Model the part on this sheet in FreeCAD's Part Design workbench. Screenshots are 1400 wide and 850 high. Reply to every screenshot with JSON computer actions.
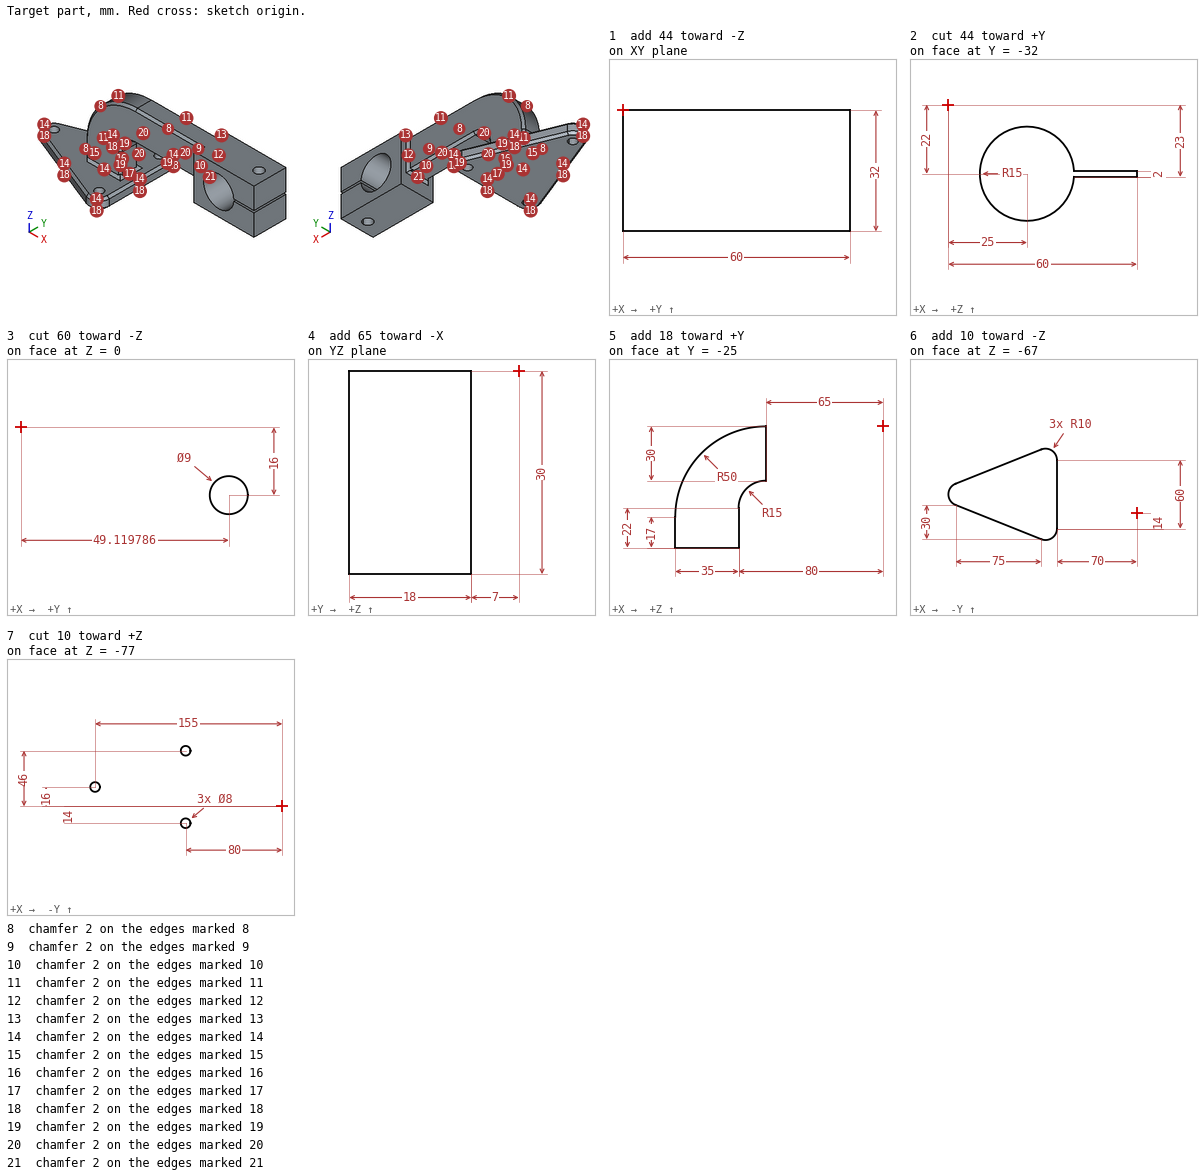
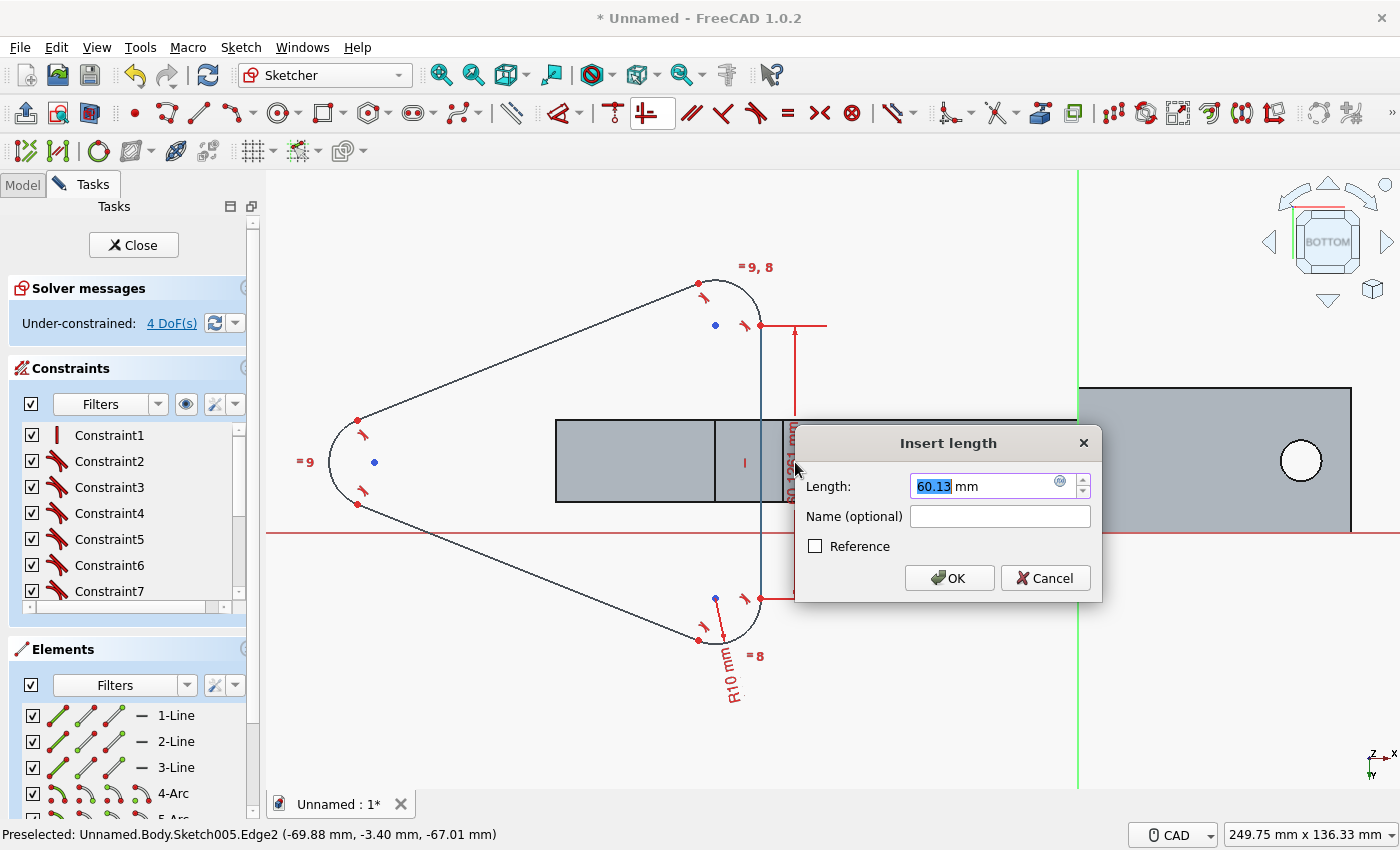
{"action": "type", "text": "60"}
{"action": "key", "text": "Return"}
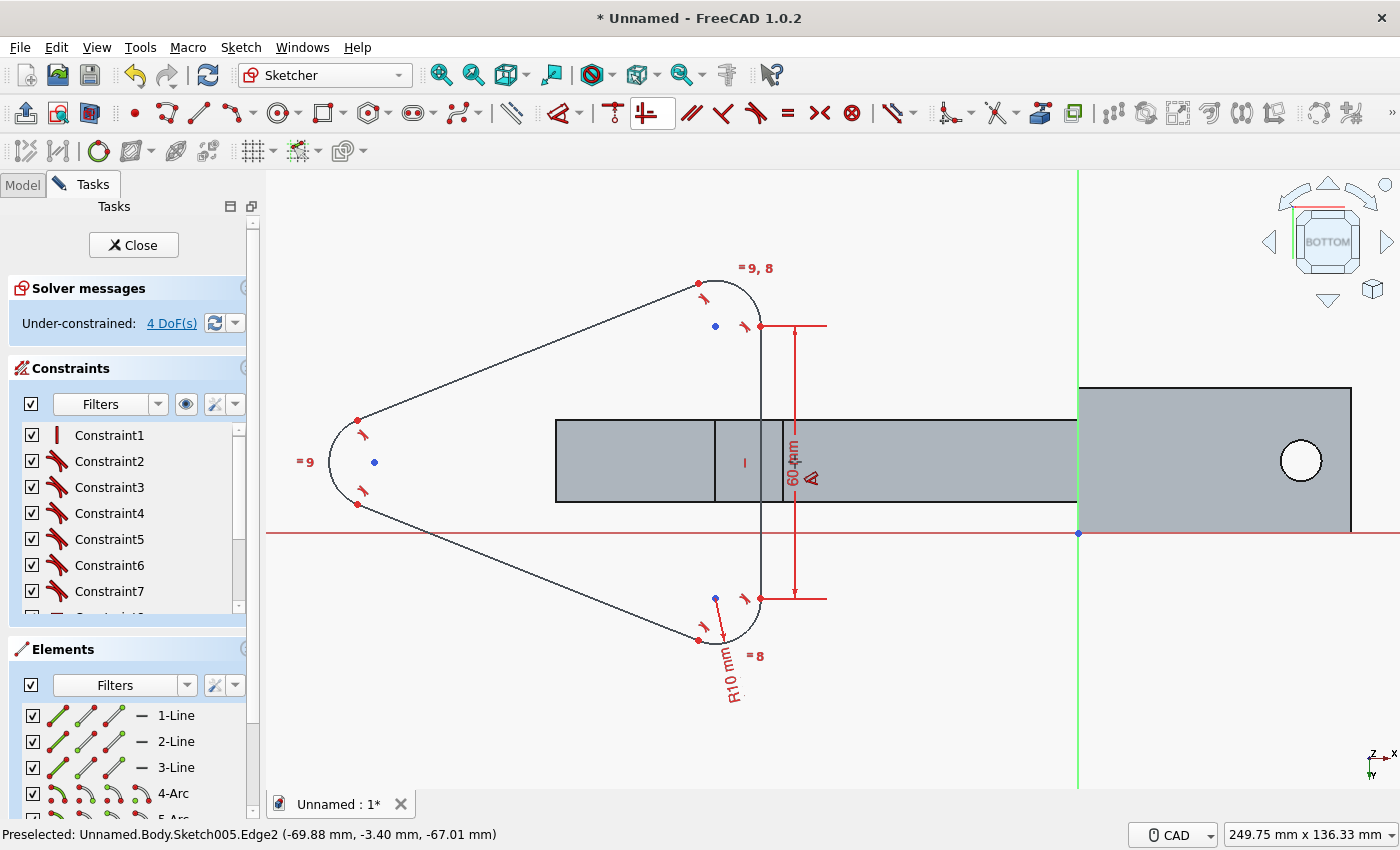
{"action": "left_click", "coordinate": [761, 599]}
{"action": "left_click", "coordinate": [920, 633]}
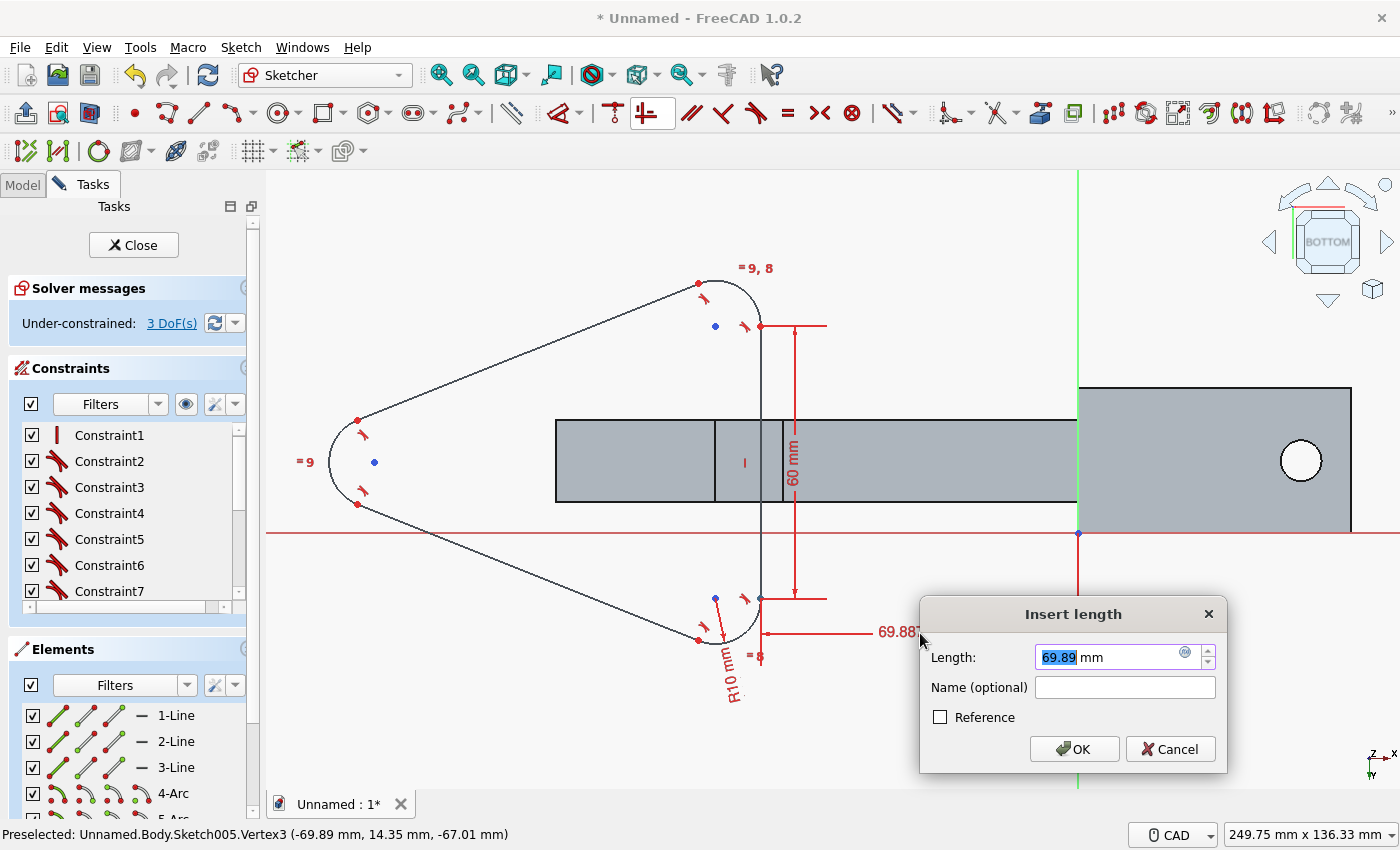
{"action": "type", "text": "70"}
{"action": "key", "text": "Return"}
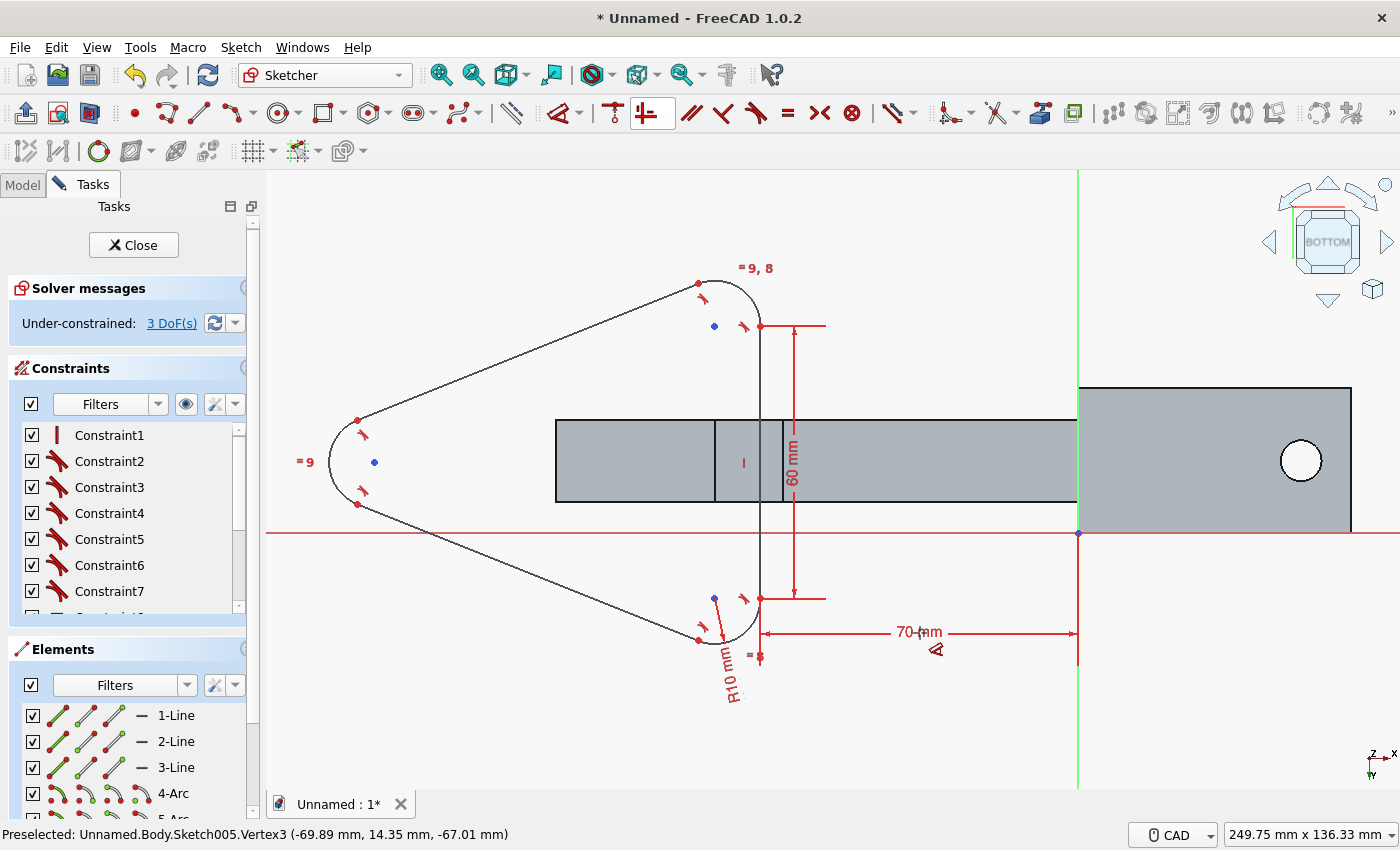
{"action": "left_click", "coordinate": [760, 599]}
{"action": "left_click", "coordinate": [1112, 566]}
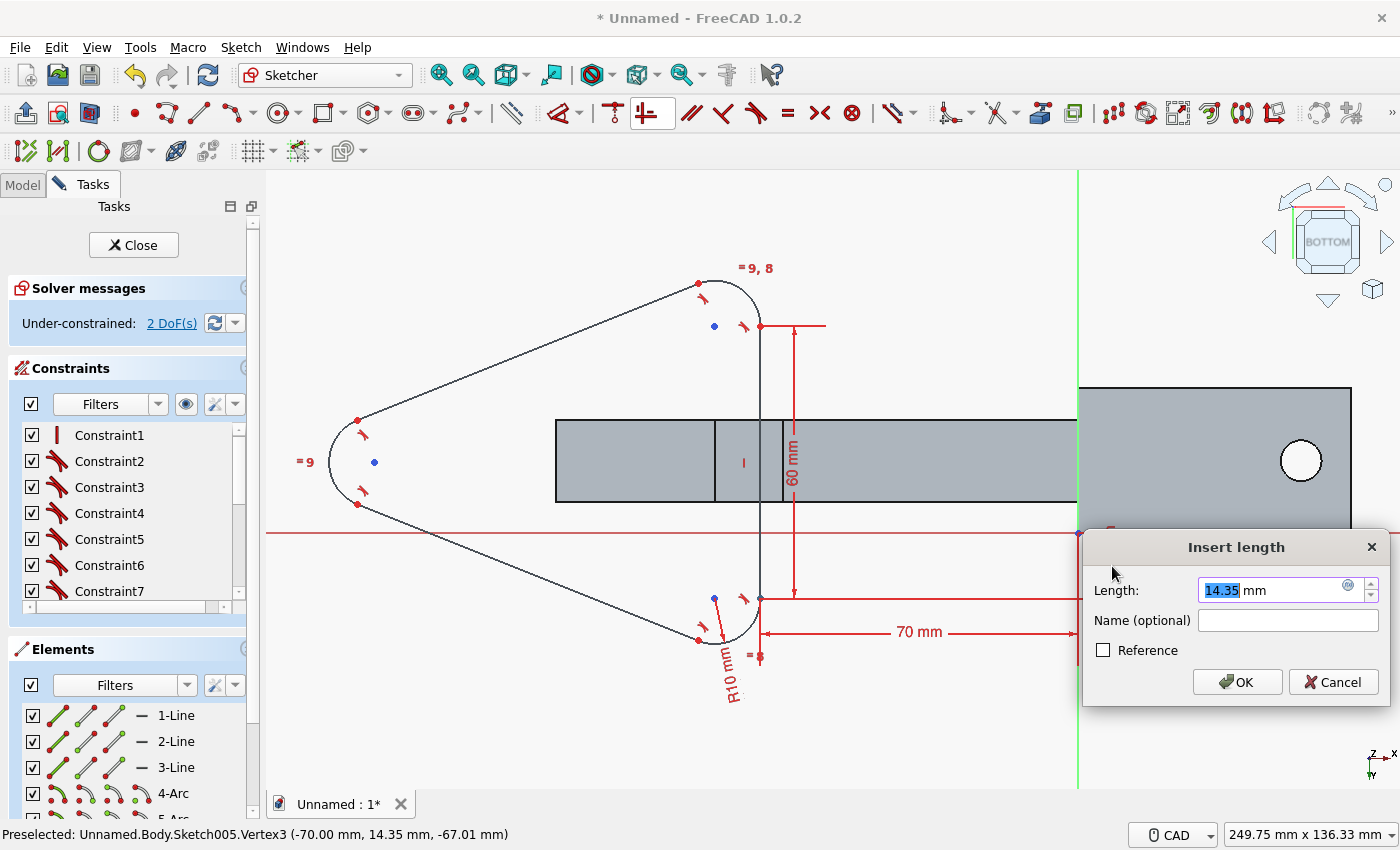
{"action": "type", "text": "14"}
{"action": "key", "text": "Return"}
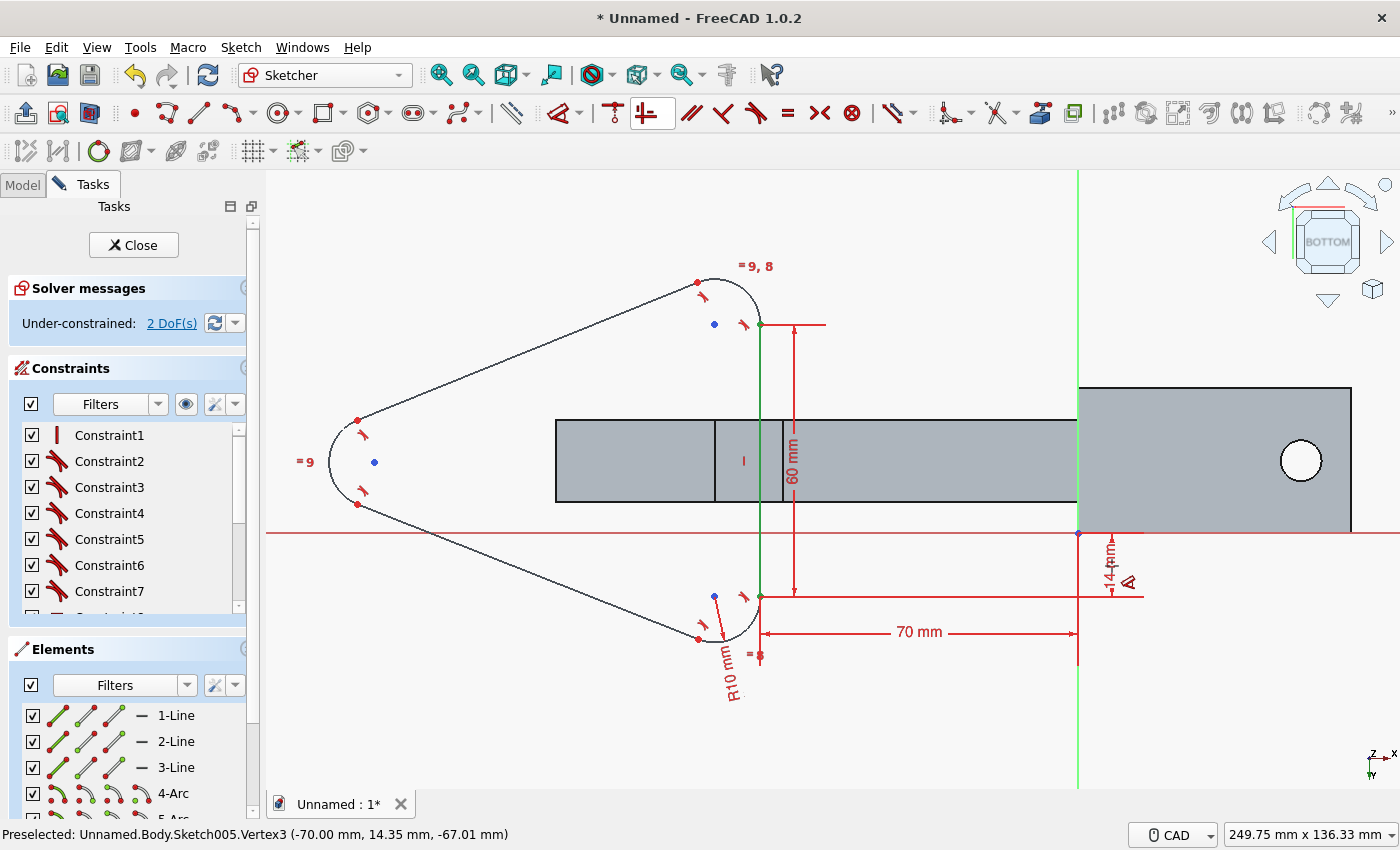
{"action": "left_click", "coordinate": [460, 545]}
{"action": "left_click", "coordinate": [528, 673]}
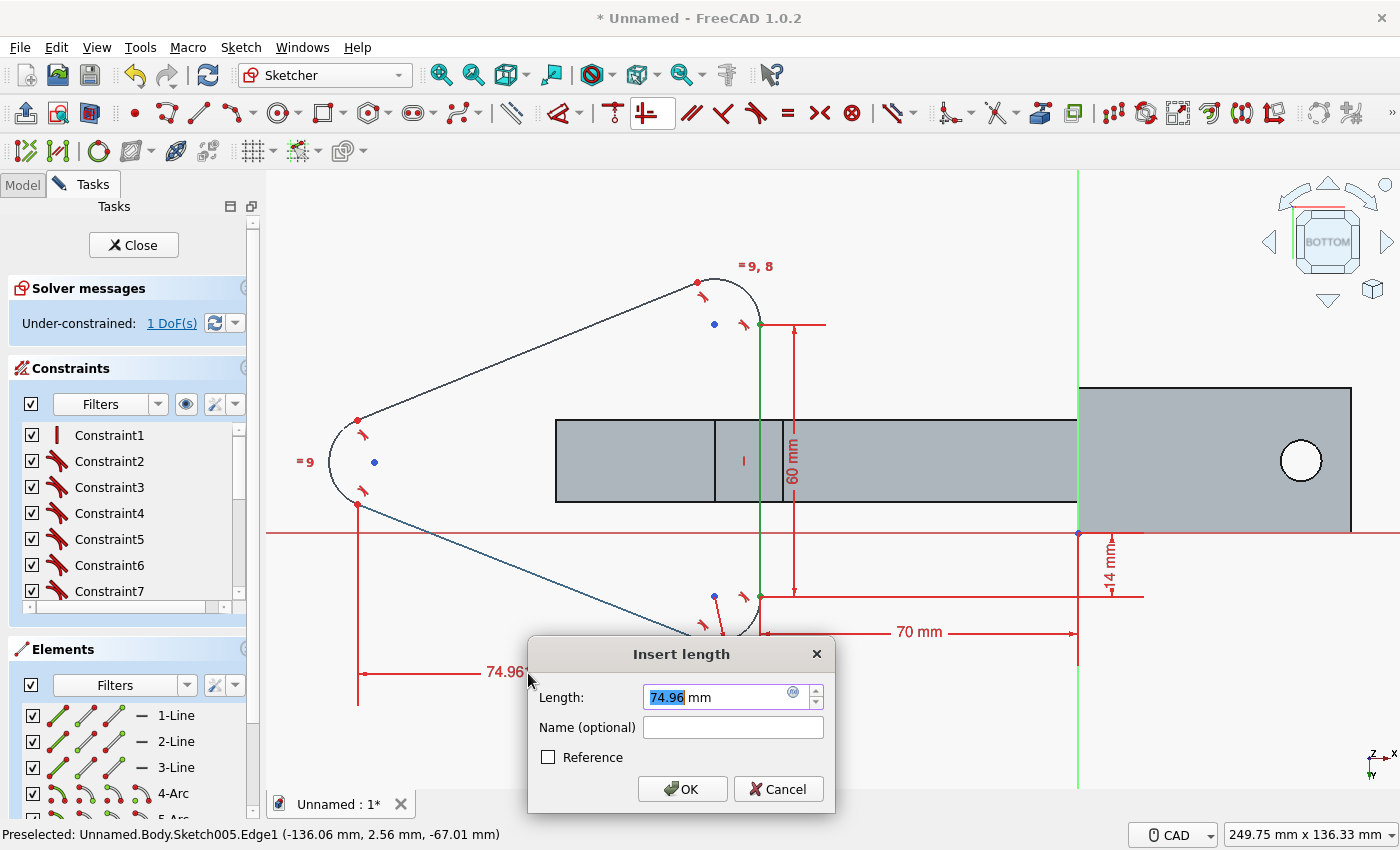
{"action": "type", "text": "75"}
{"action": "key", "text": "Return"}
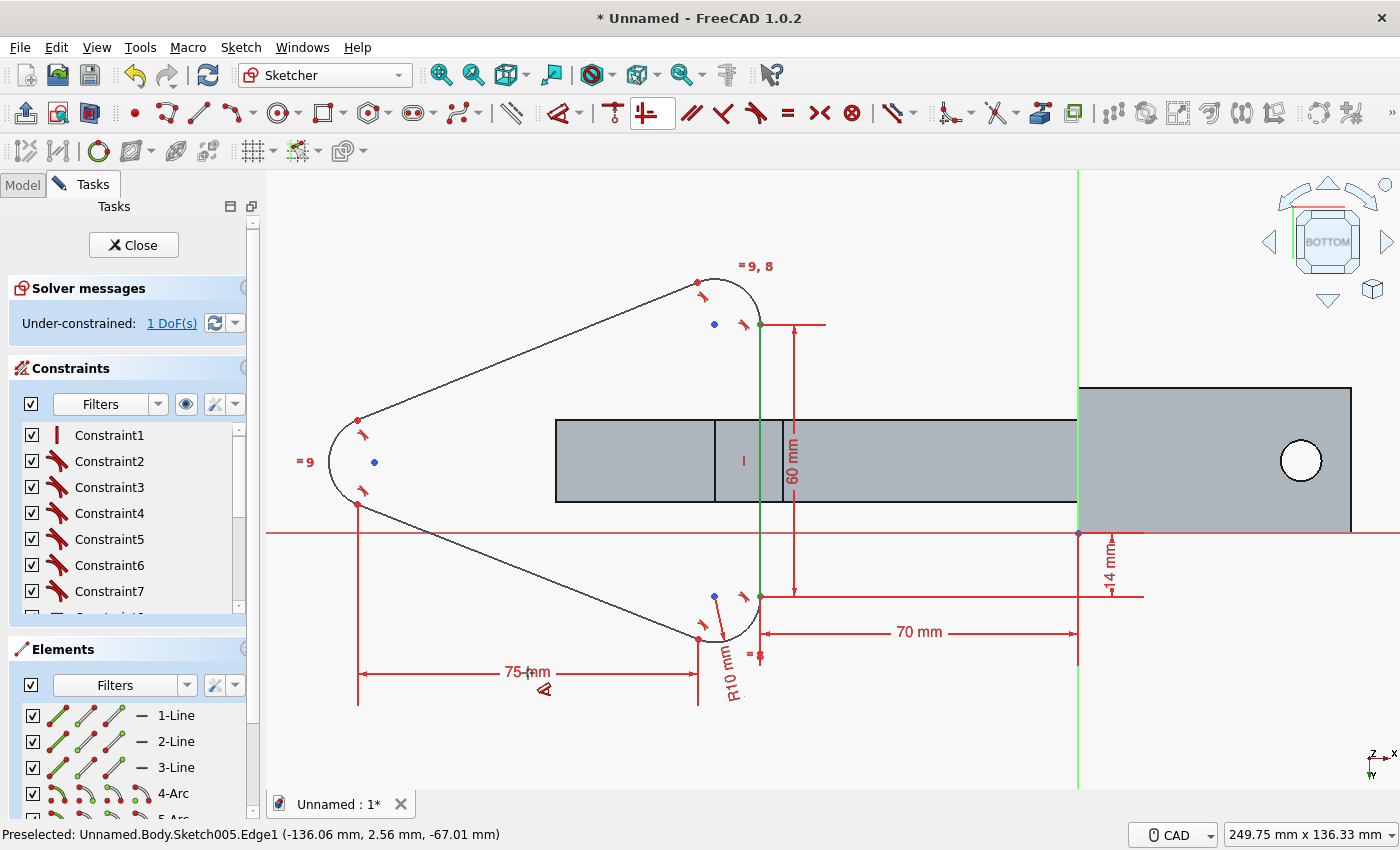
{"action": "left_click", "coordinate": [460, 545]}
{"action": "left_click", "coordinate": [324, 572]}